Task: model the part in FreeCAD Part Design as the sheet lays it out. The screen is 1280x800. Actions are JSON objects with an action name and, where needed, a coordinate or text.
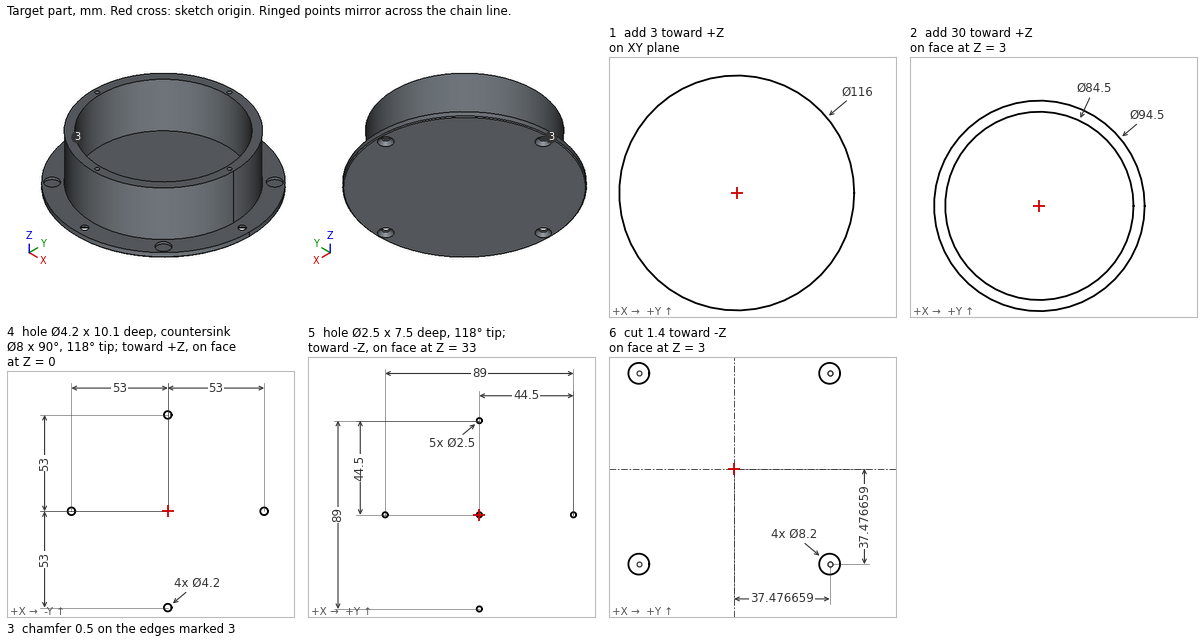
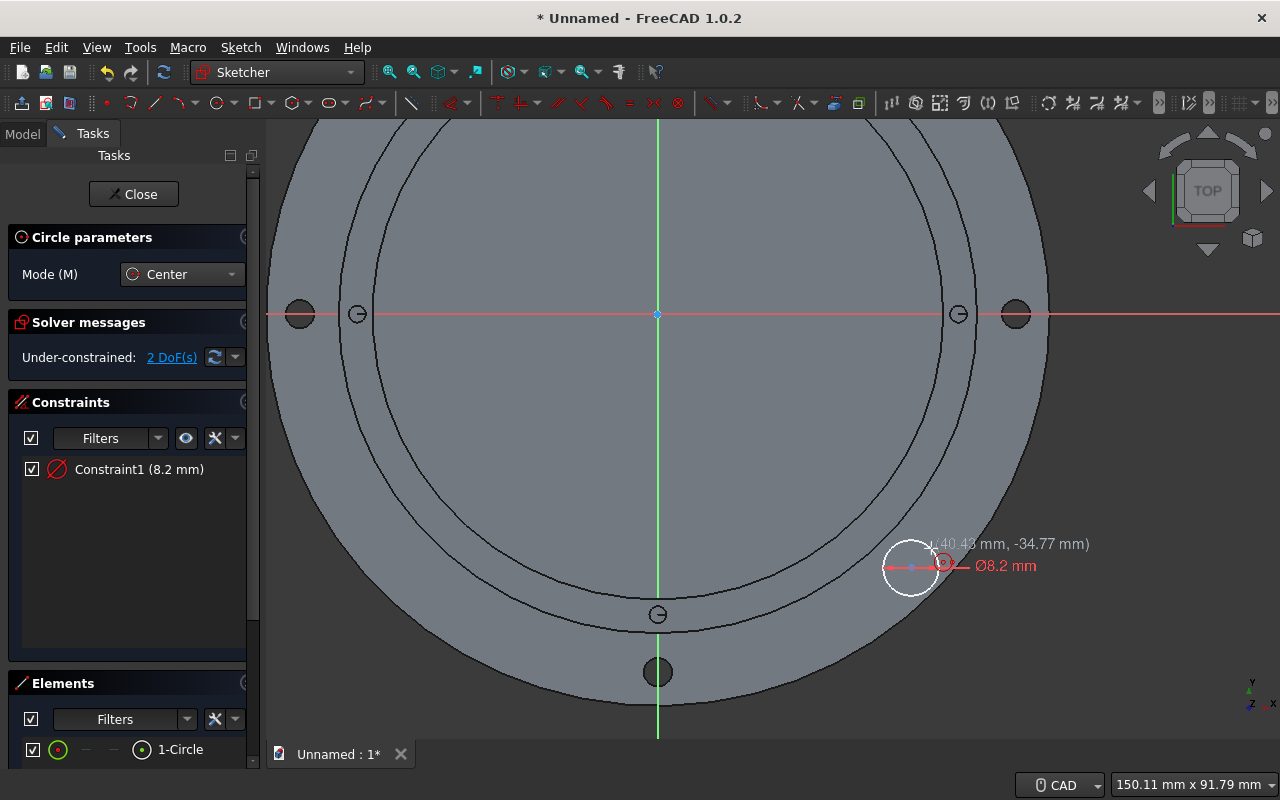
{"action": "scroll", "coordinate": [799, 663], "scroll_direction": "down", "scroll_amount": 2}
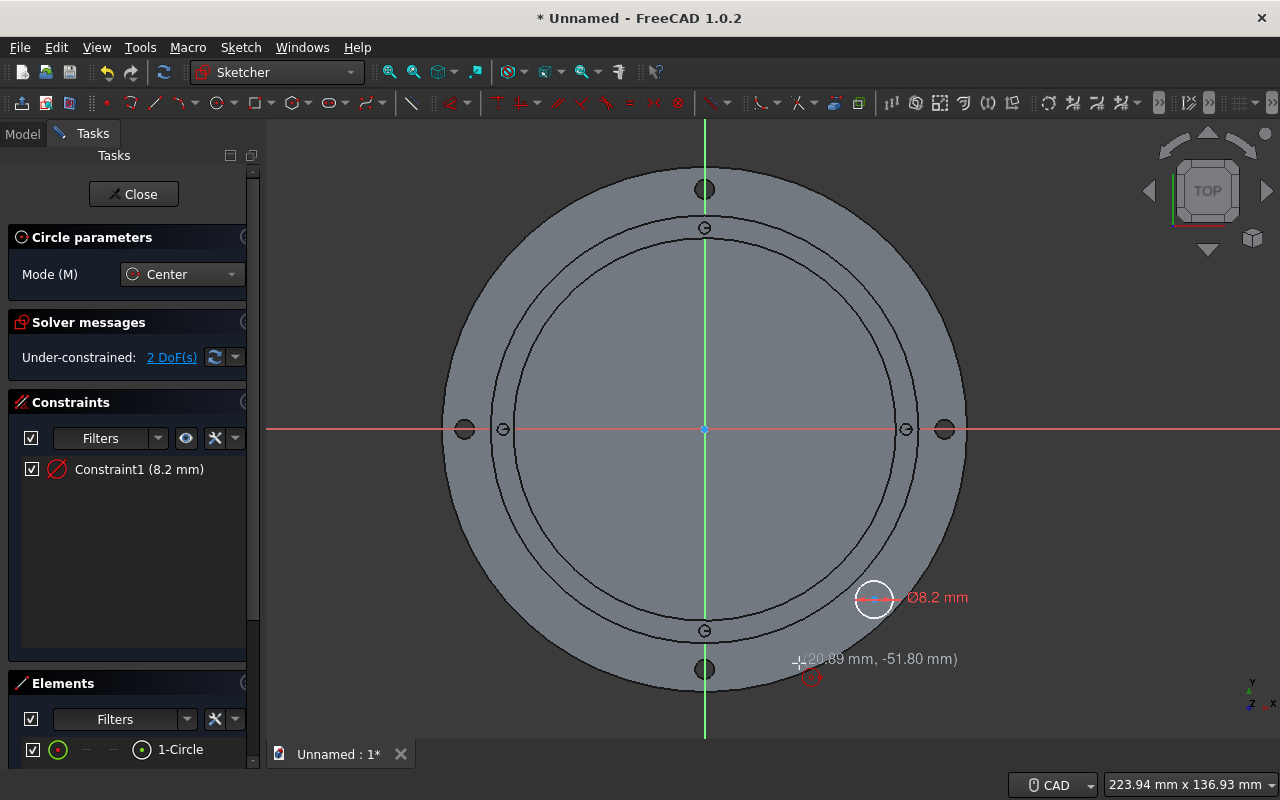
{"action": "scroll", "coordinate": [874, 260], "scroll_direction": "up", "scroll_amount": 2}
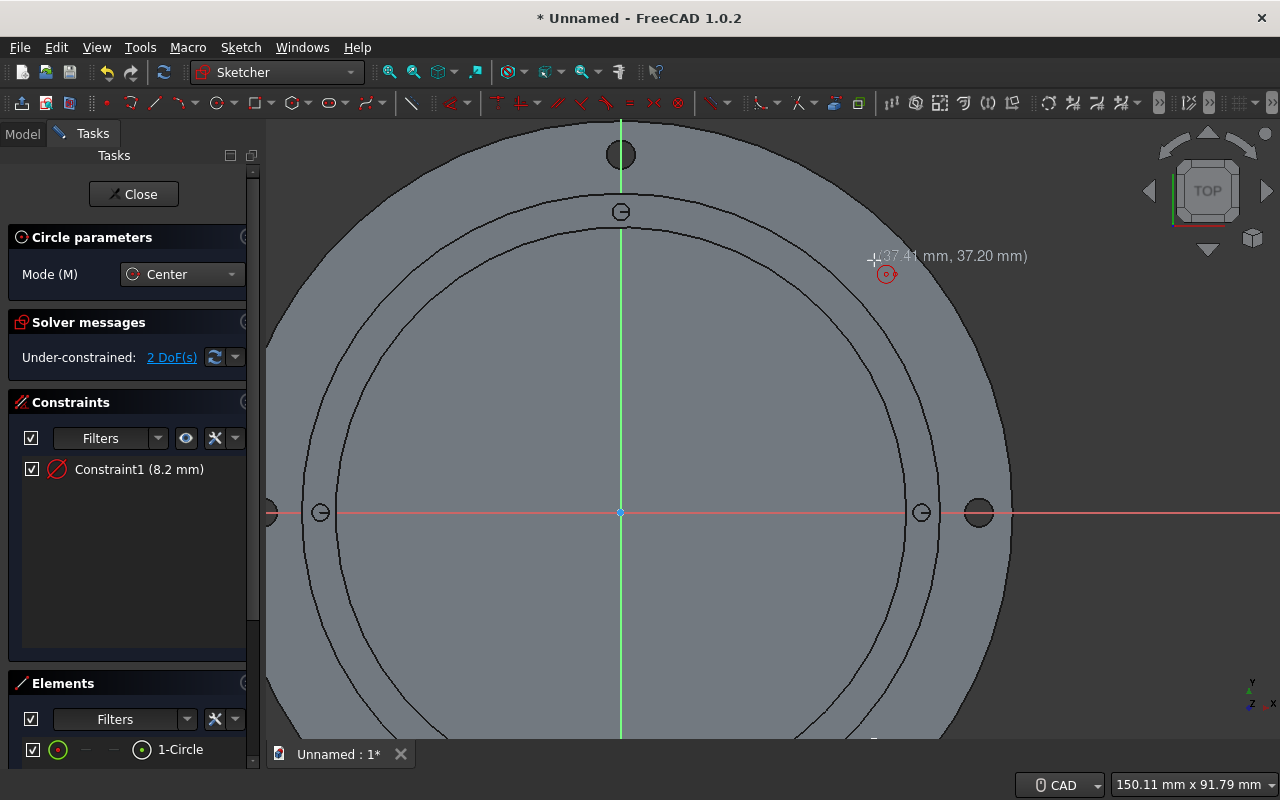
{"action": "left_click", "coordinate": [874, 260]}
{"action": "mouse_move", "coordinate": [894, 240]}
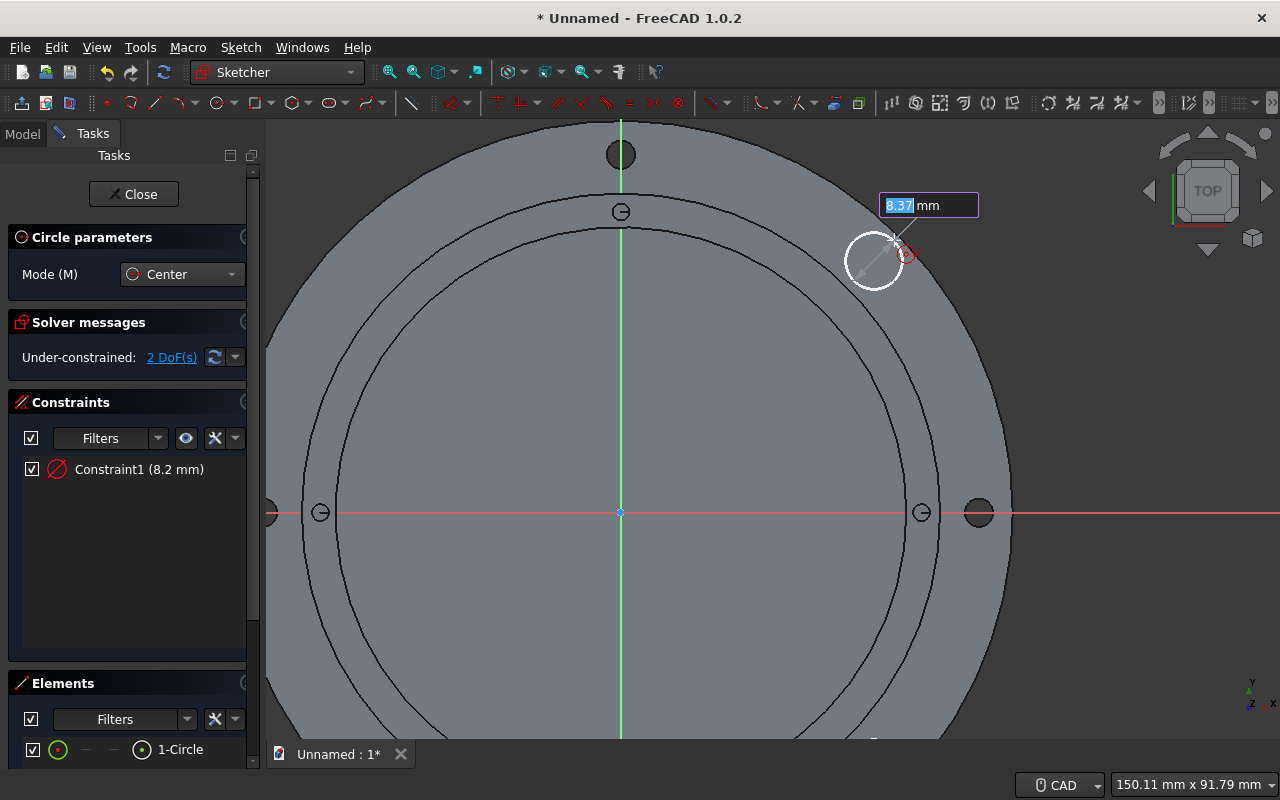
{"action": "type", "text": "8.2"}
{"action": "key", "text": "Return"}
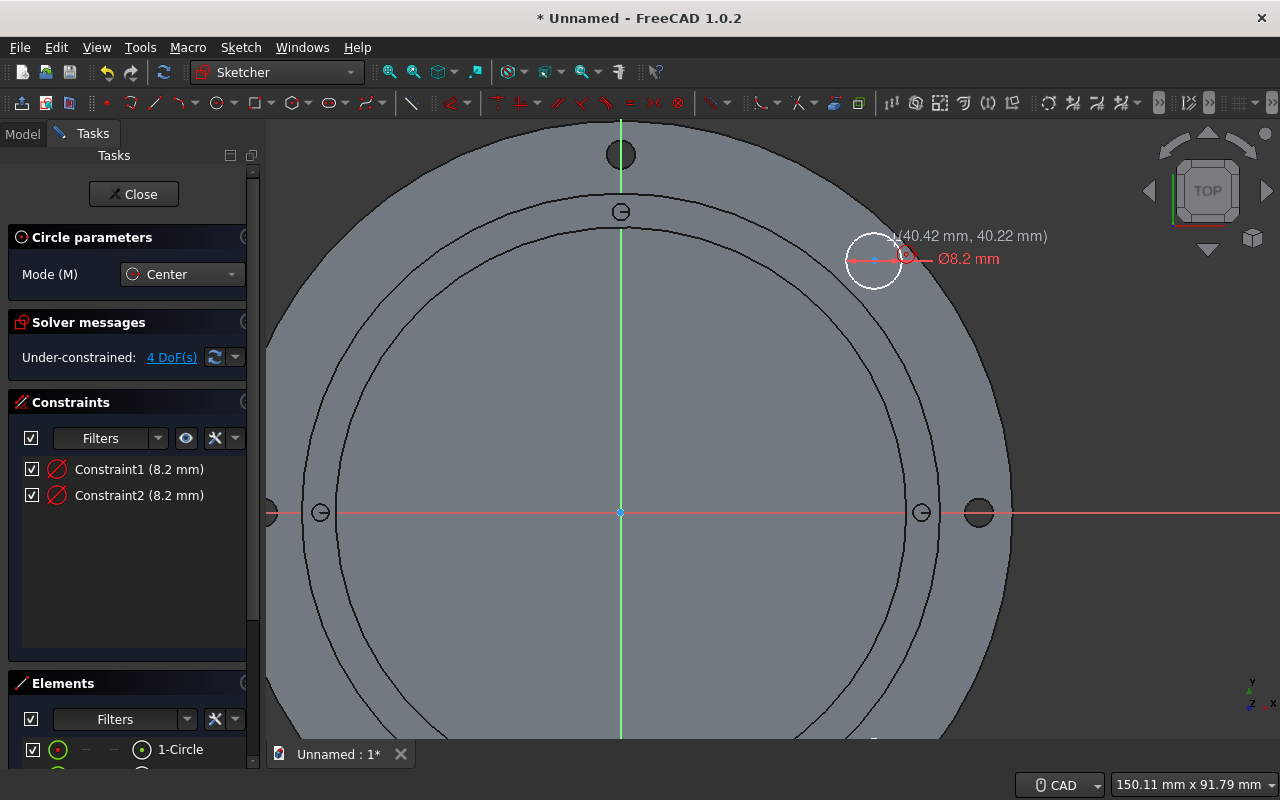
{"action": "left_click", "coordinate": [368, 260]}
{"action": "mouse_move", "coordinate": [387, 240]}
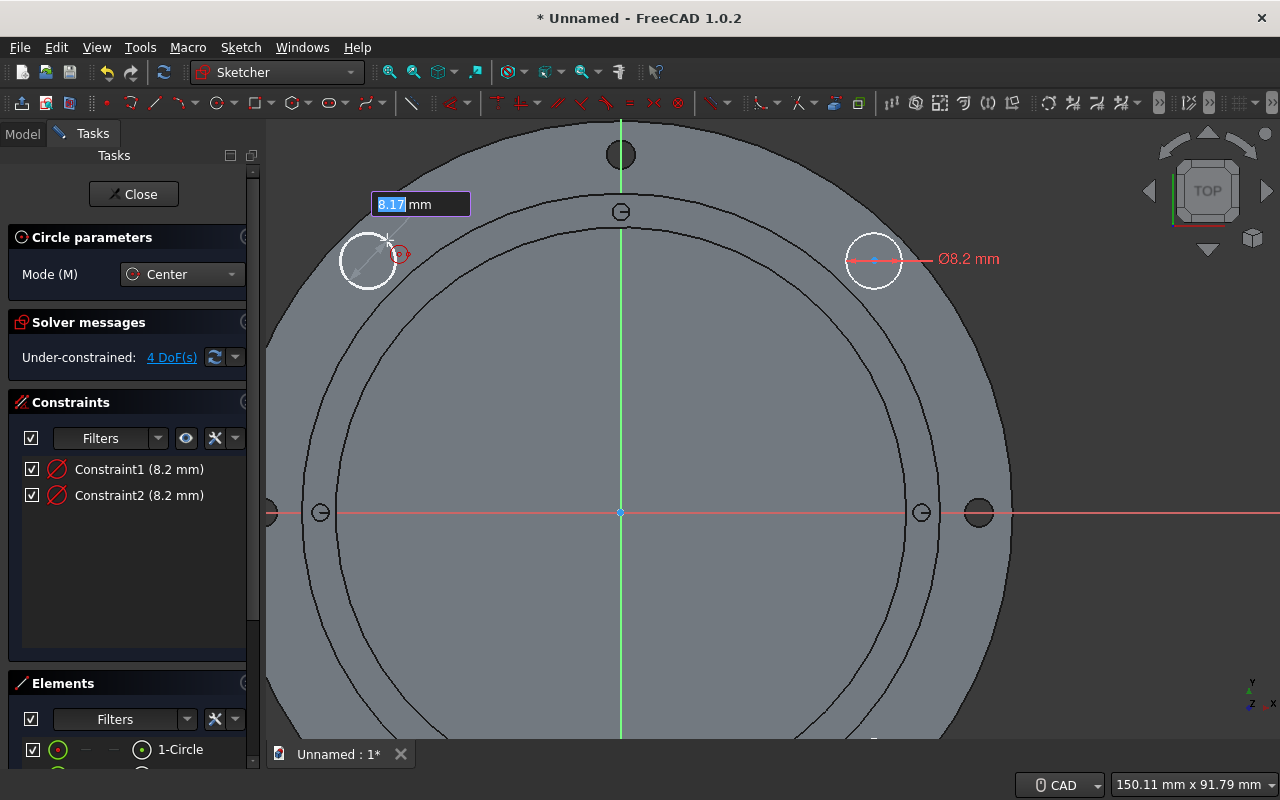
{"action": "type", "text": "8.2"}
{"action": "key", "text": "Return"}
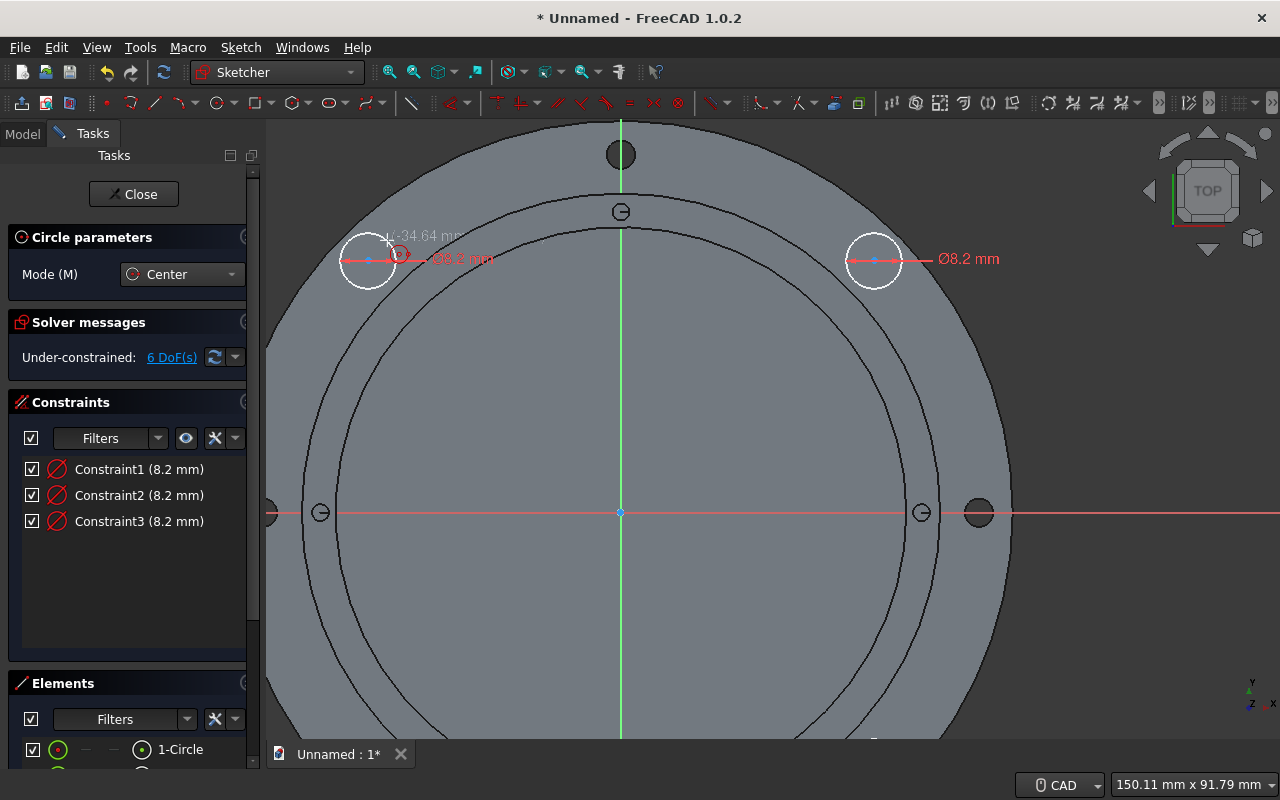
{"action": "scroll", "coordinate": [874, 259], "scroll_direction": "down", "scroll_amount": 2}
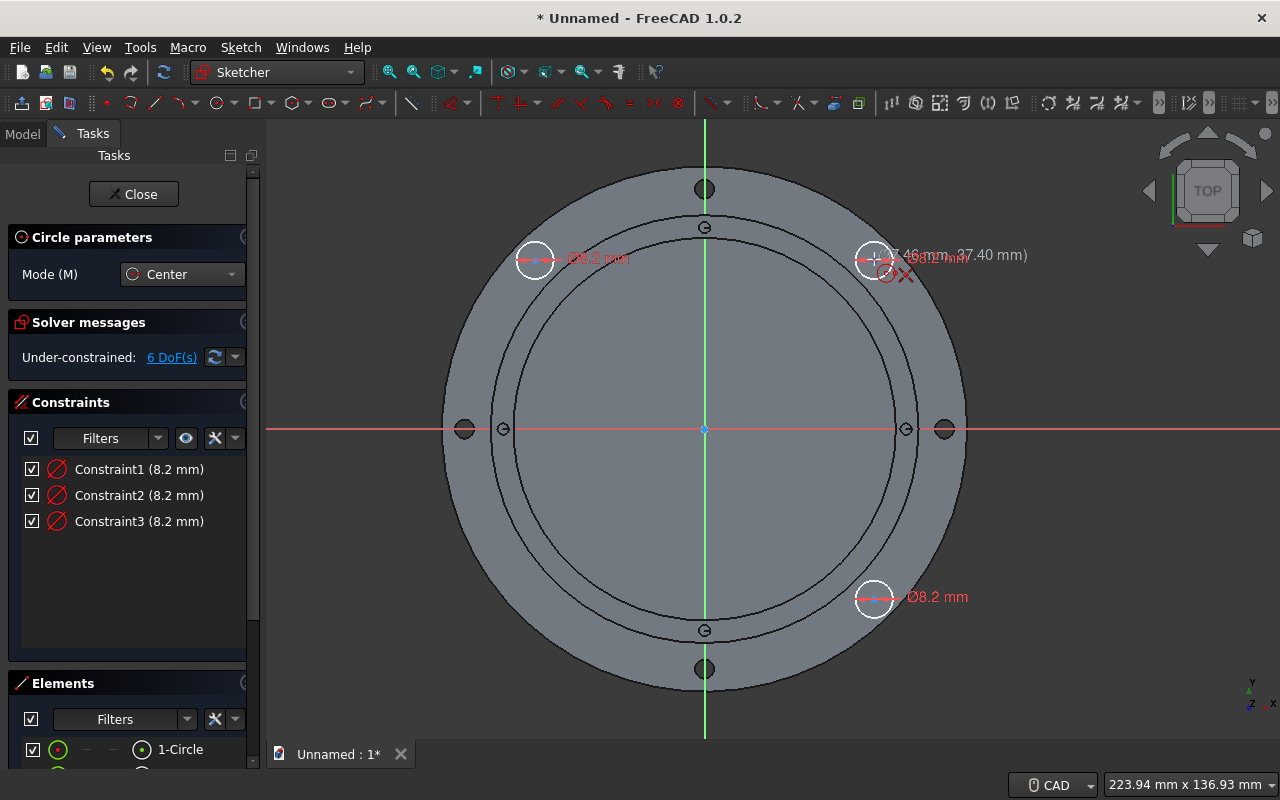
{"action": "scroll", "coordinate": [535, 599], "scroll_direction": "up", "scroll_amount": 2}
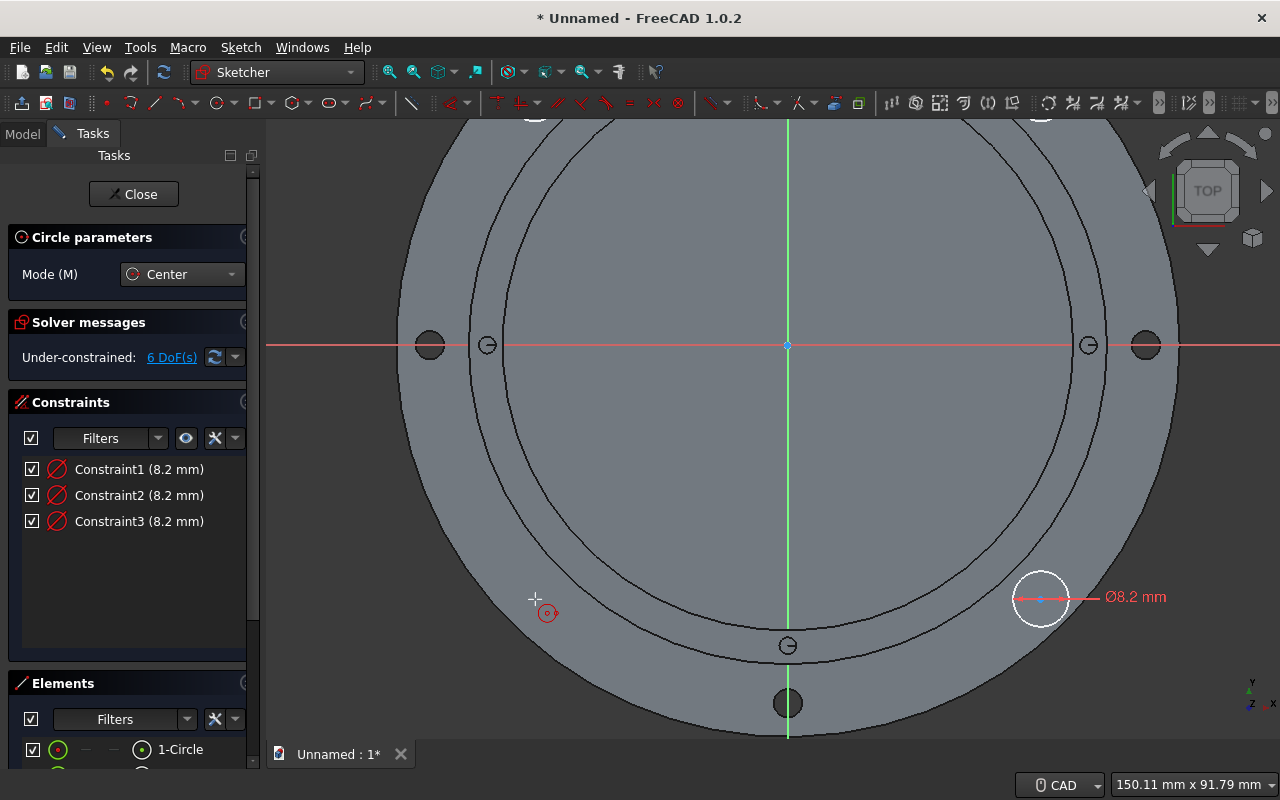
{"action": "left_click", "coordinate": [535, 598]}
{"action": "mouse_move", "coordinate": [554, 579]}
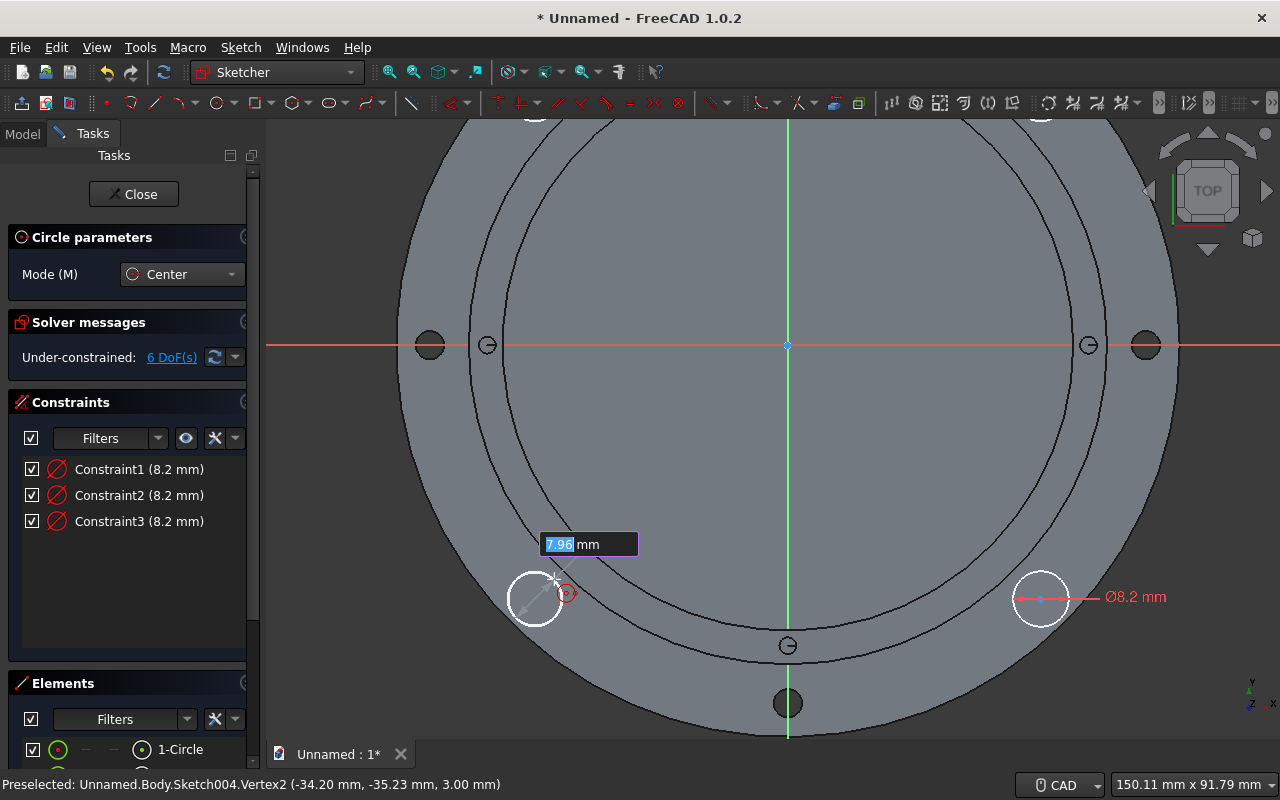
{"action": "type", "text": "8.2"}
{"action": "key", "text": "Return"}
{"action": "key", "text": "Escape"}